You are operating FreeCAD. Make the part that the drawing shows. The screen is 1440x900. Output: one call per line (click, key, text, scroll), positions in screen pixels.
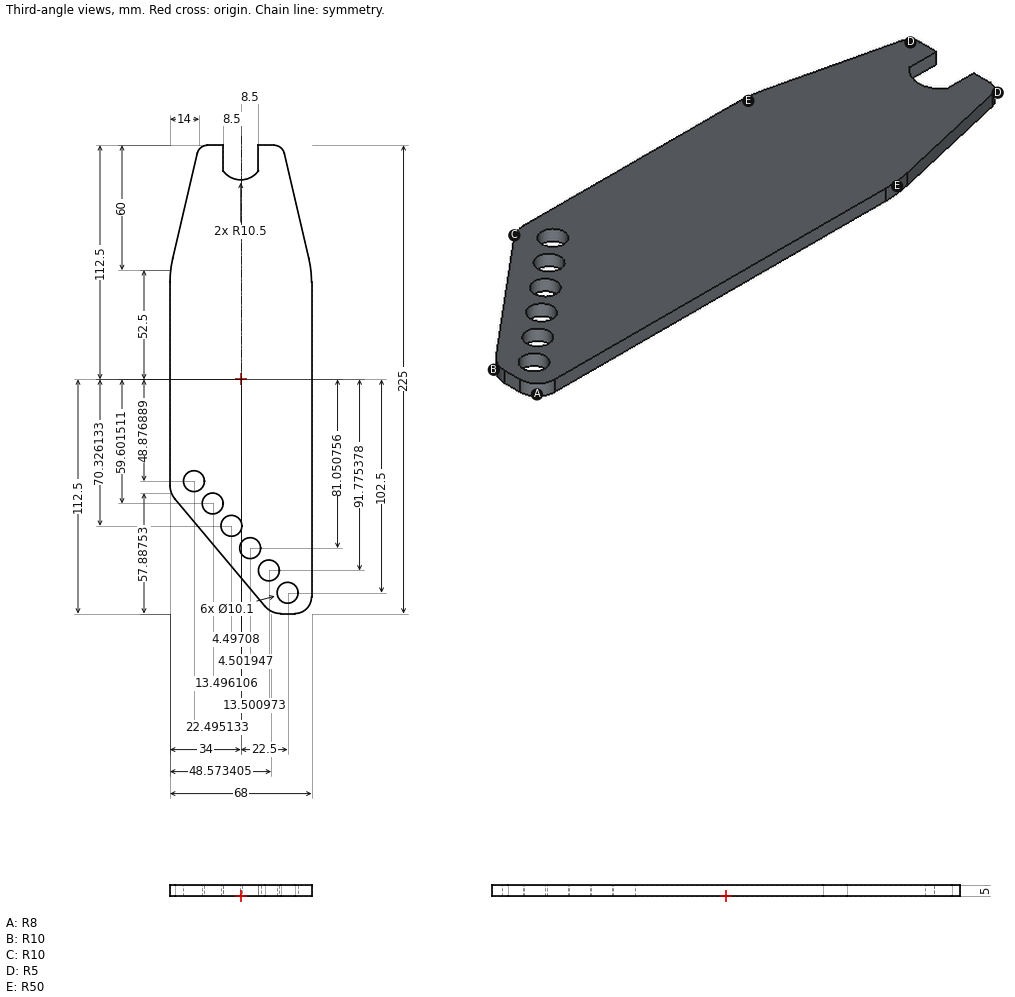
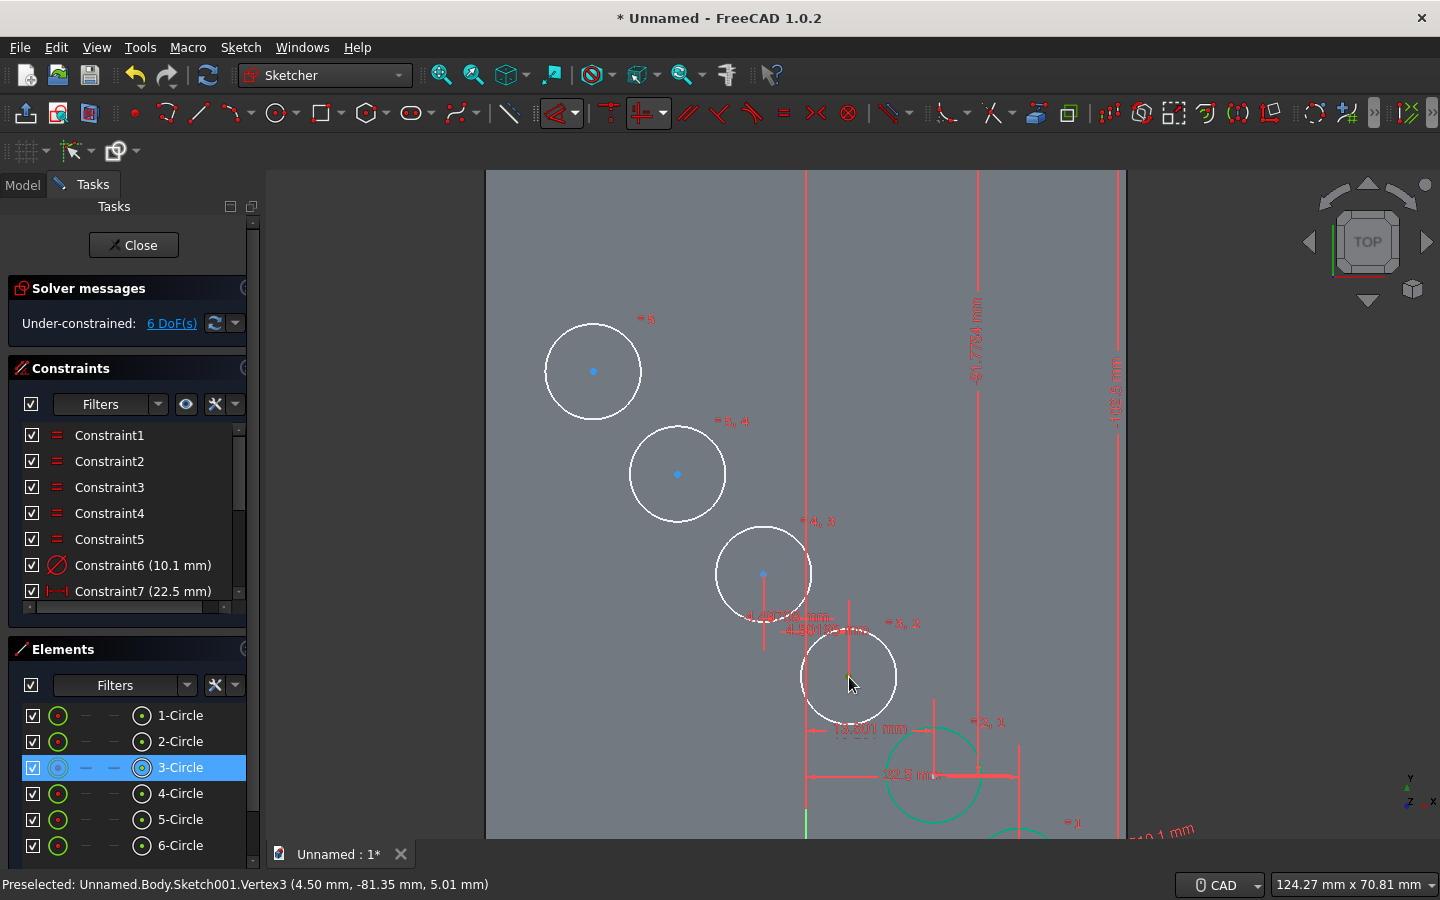
click(578, 114)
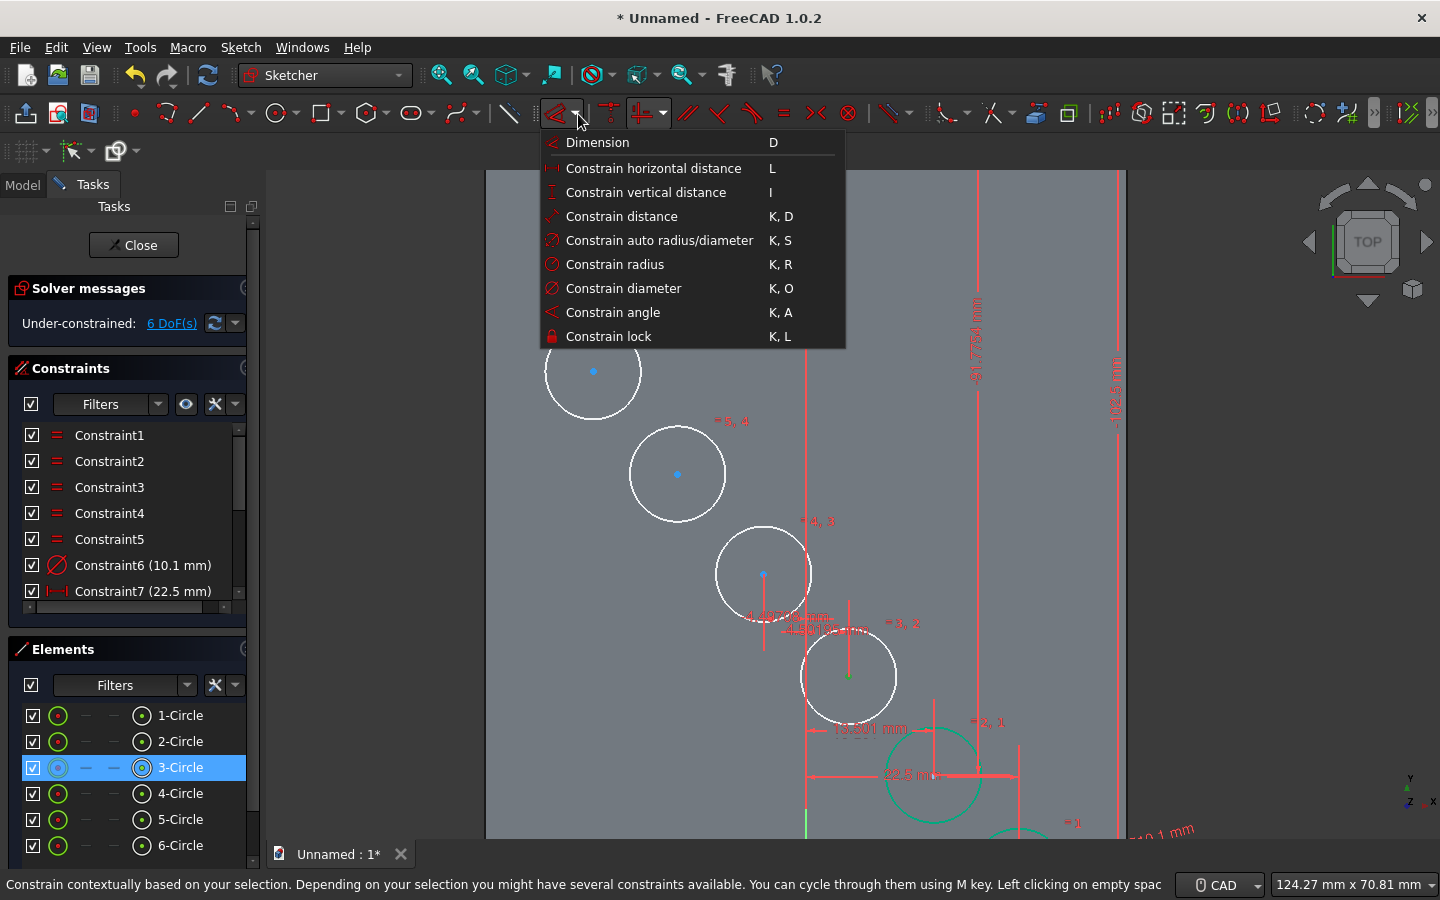
click(693, 192)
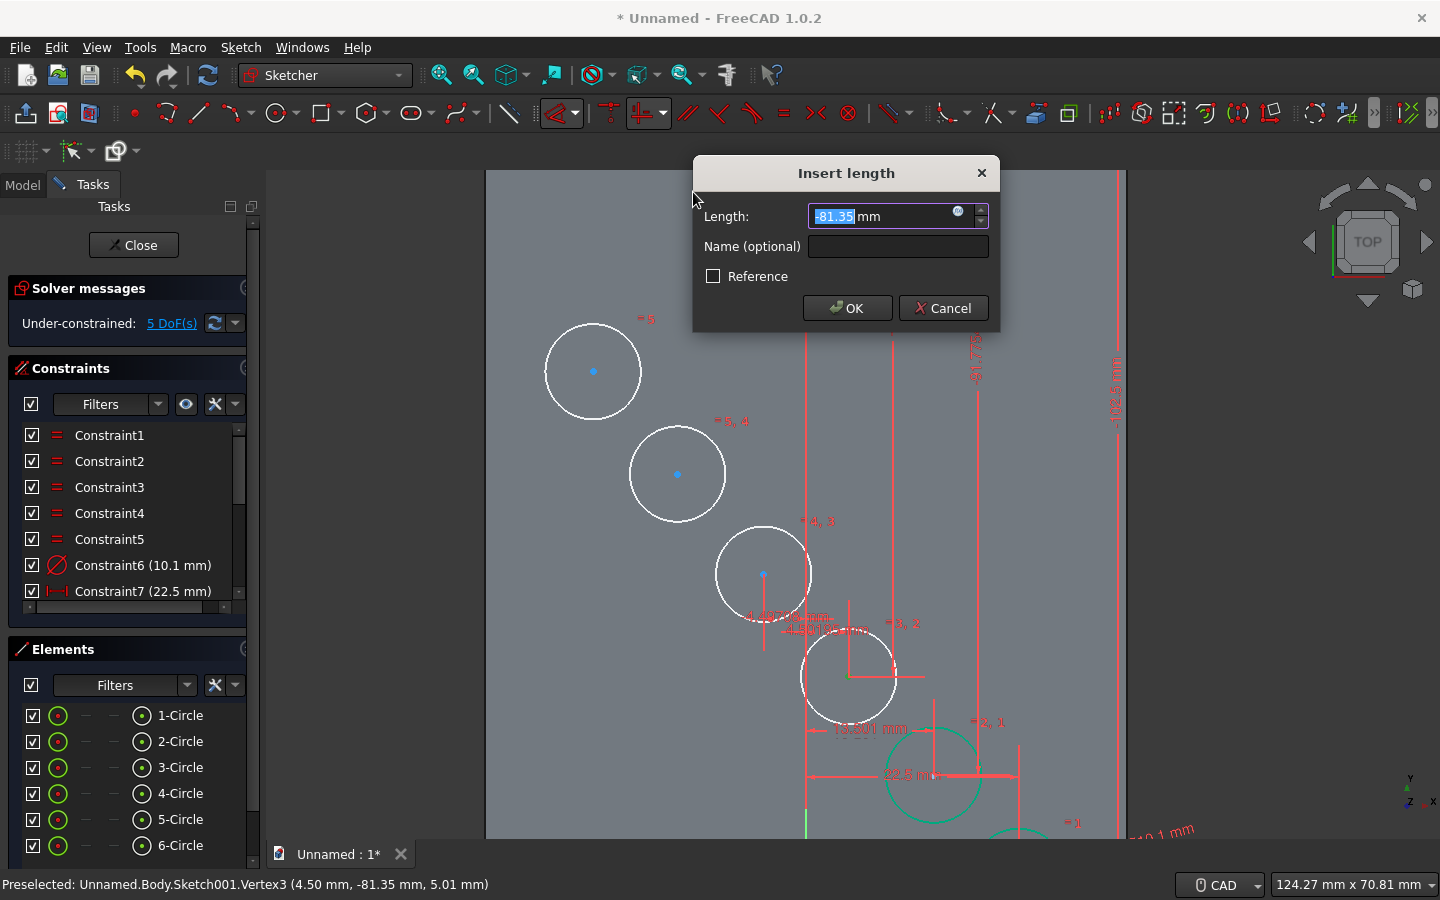
text(-81.050756)
key(Return)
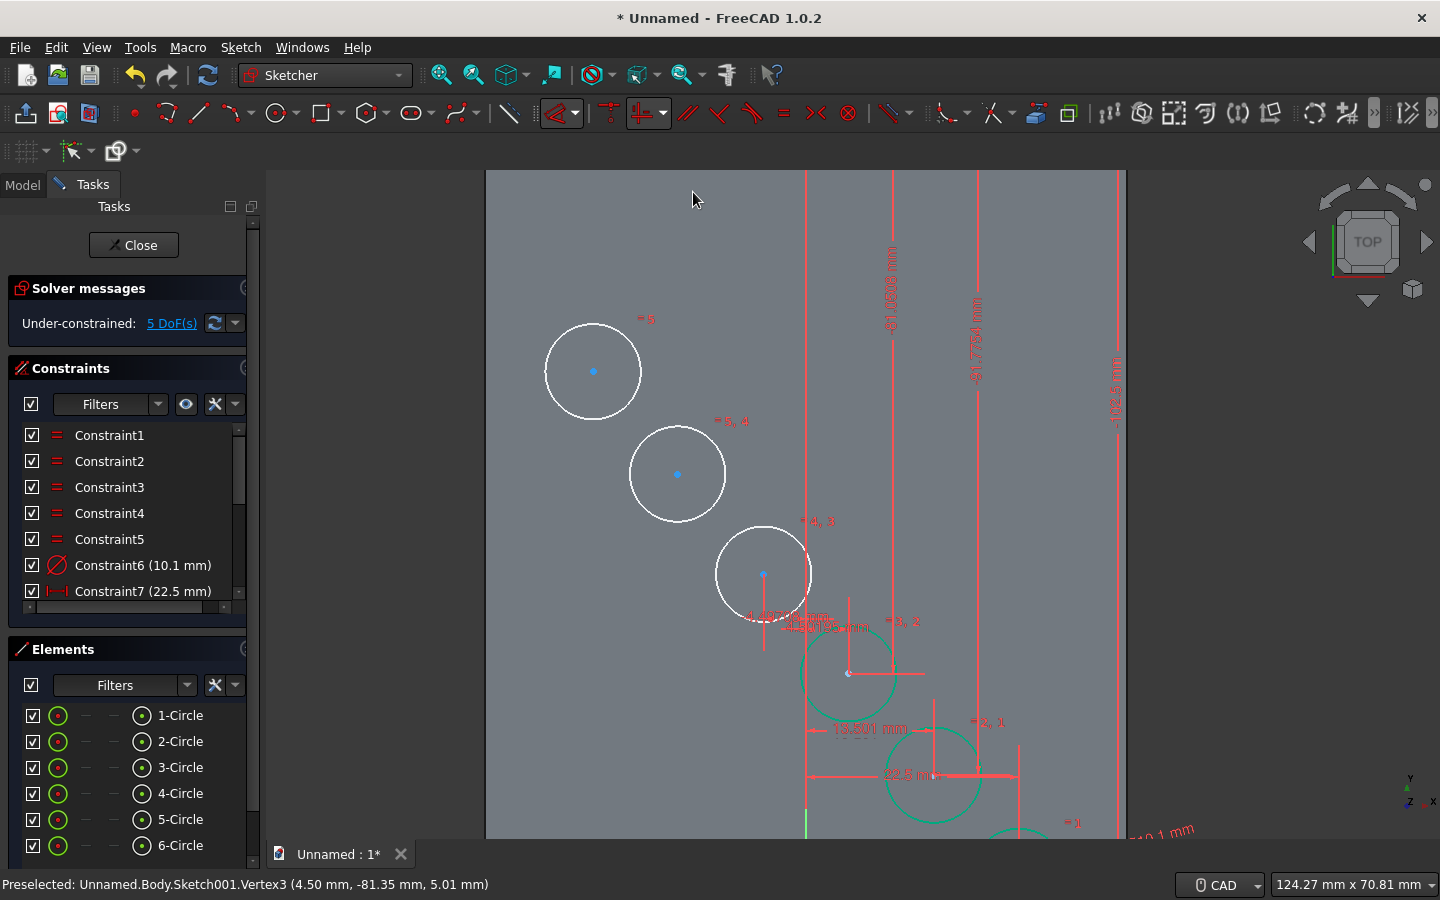
click(764, 574)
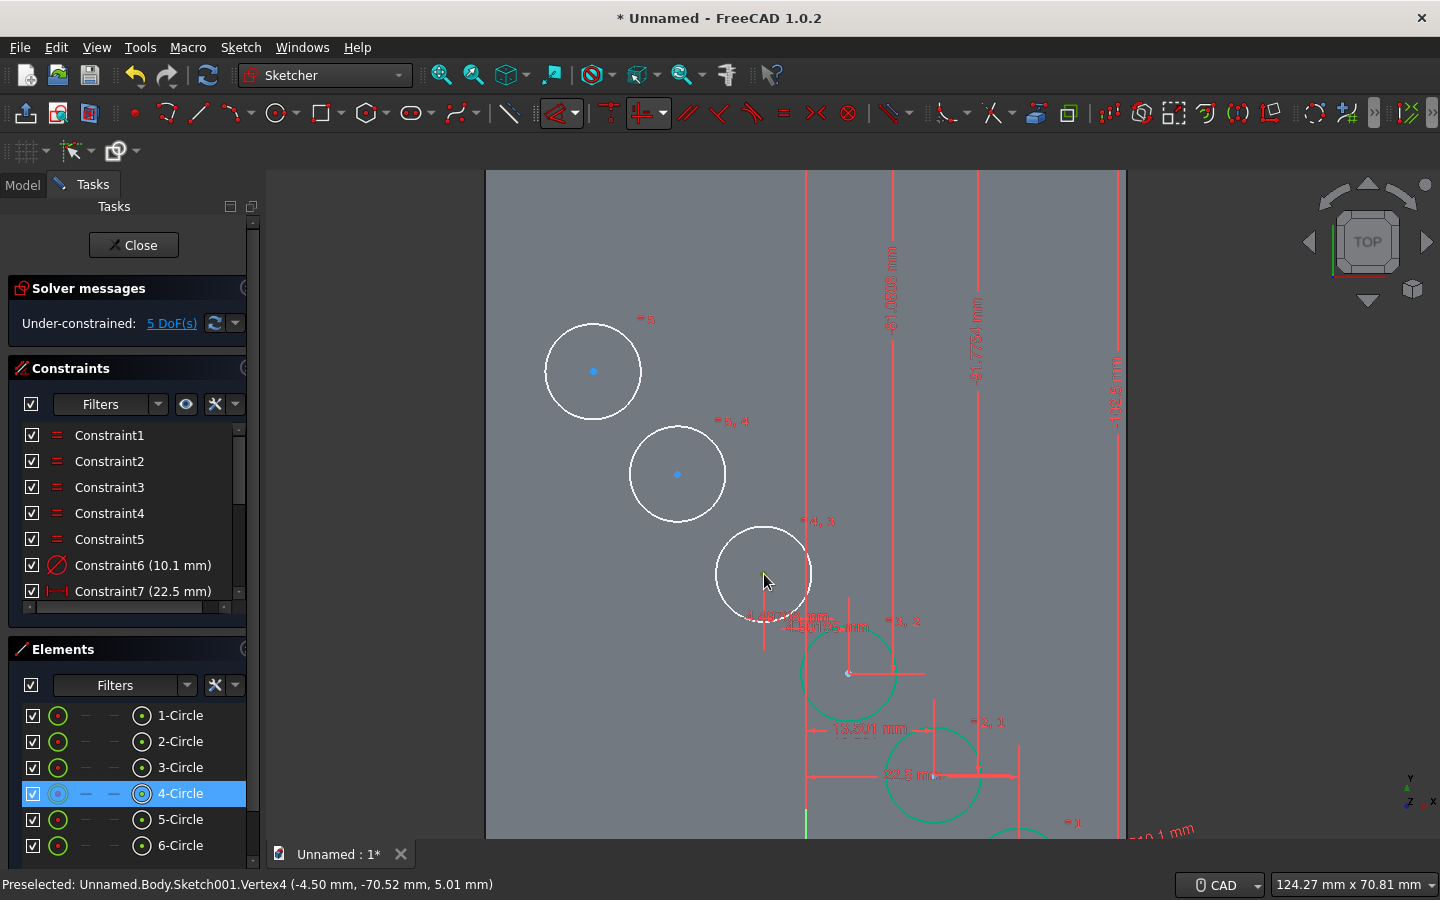
key(i)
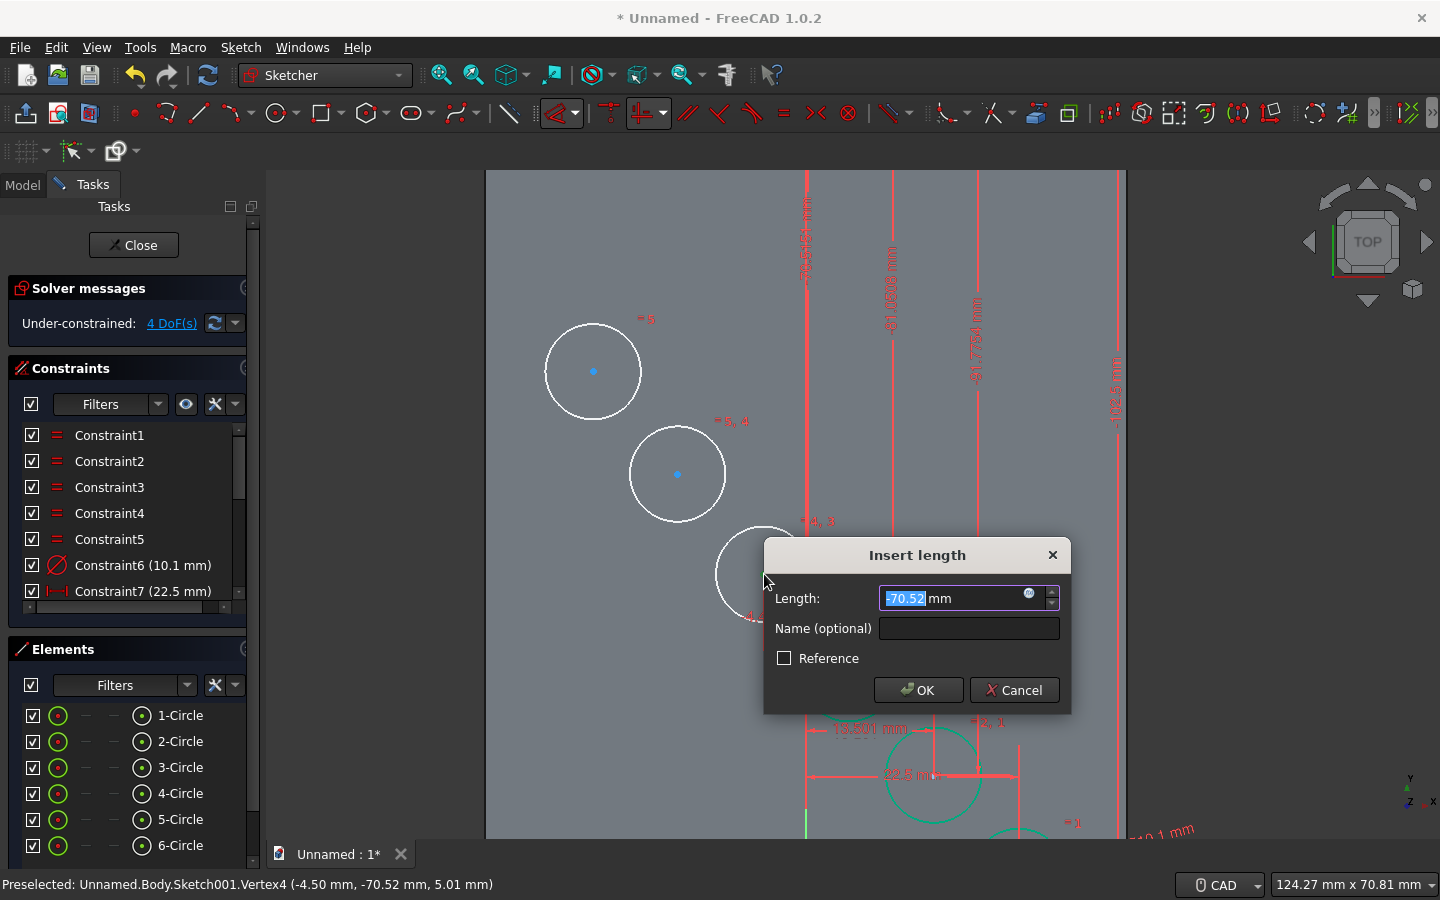
text(-70.326133)
key(Return)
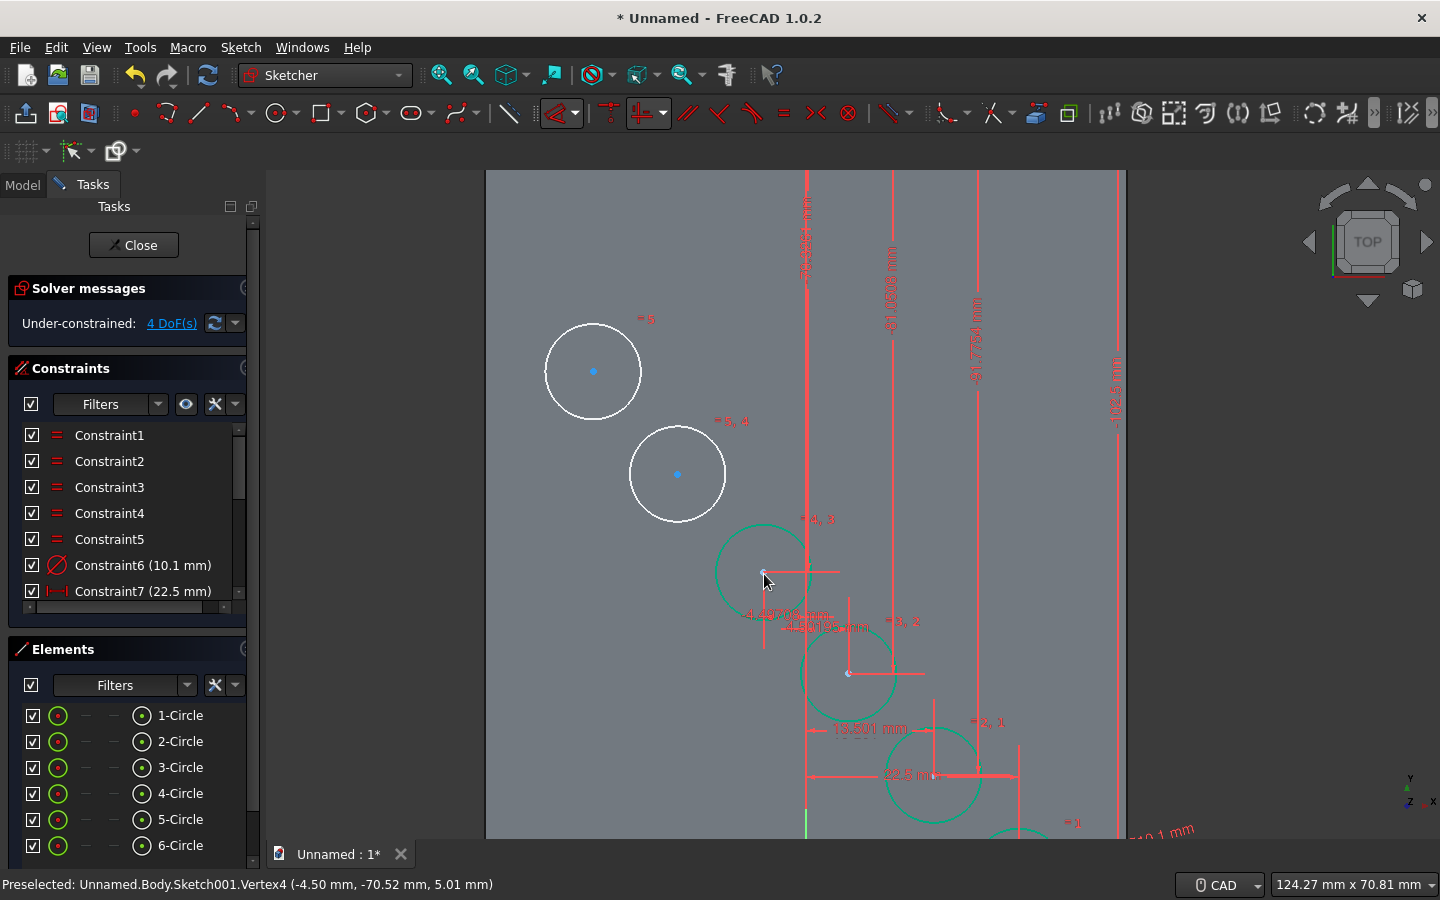
click(678, 474)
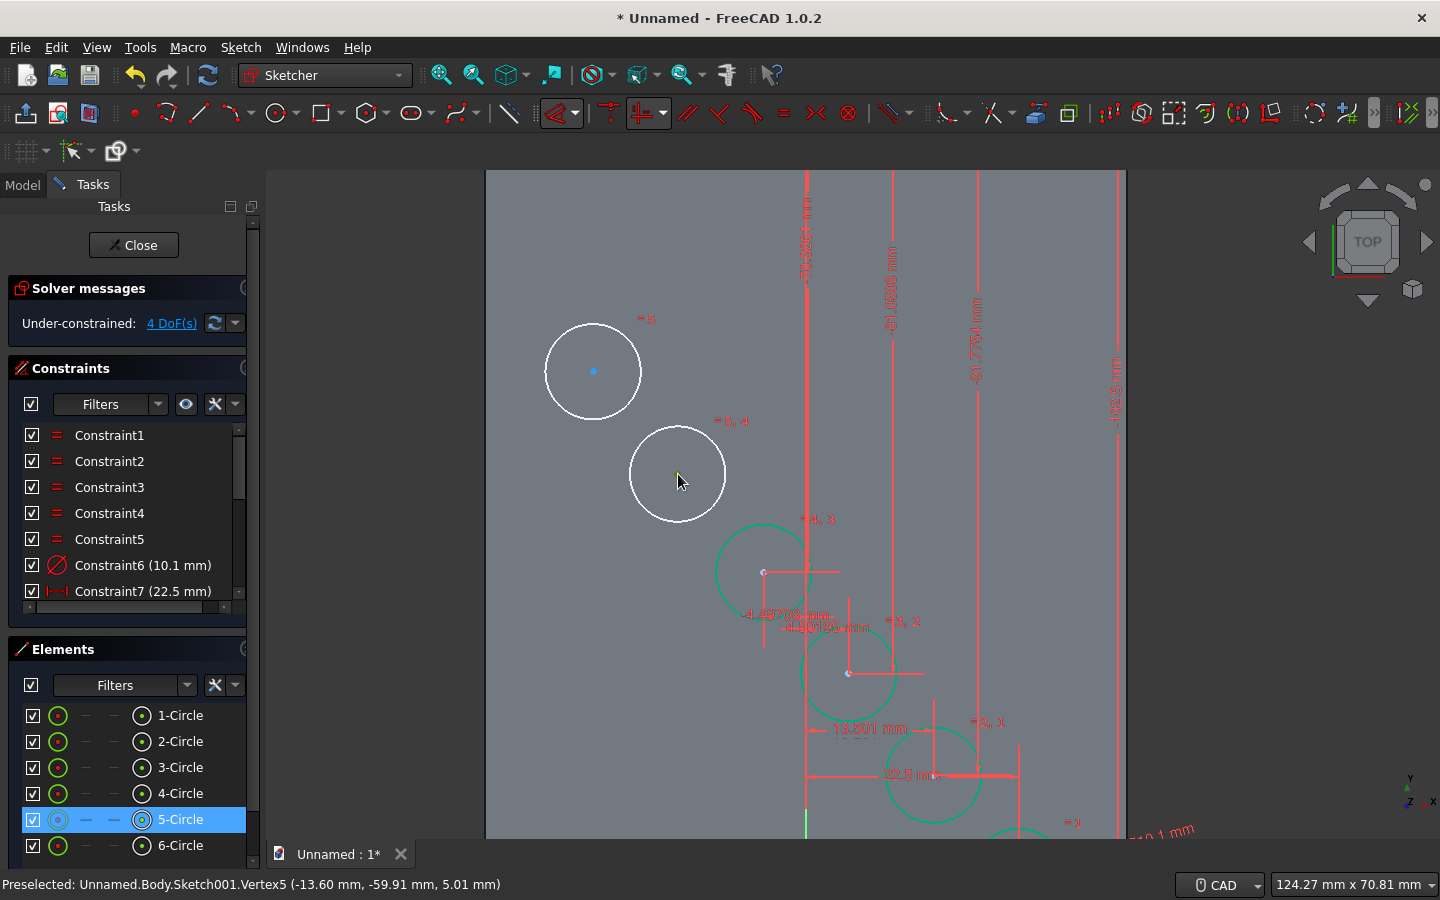
key(l)